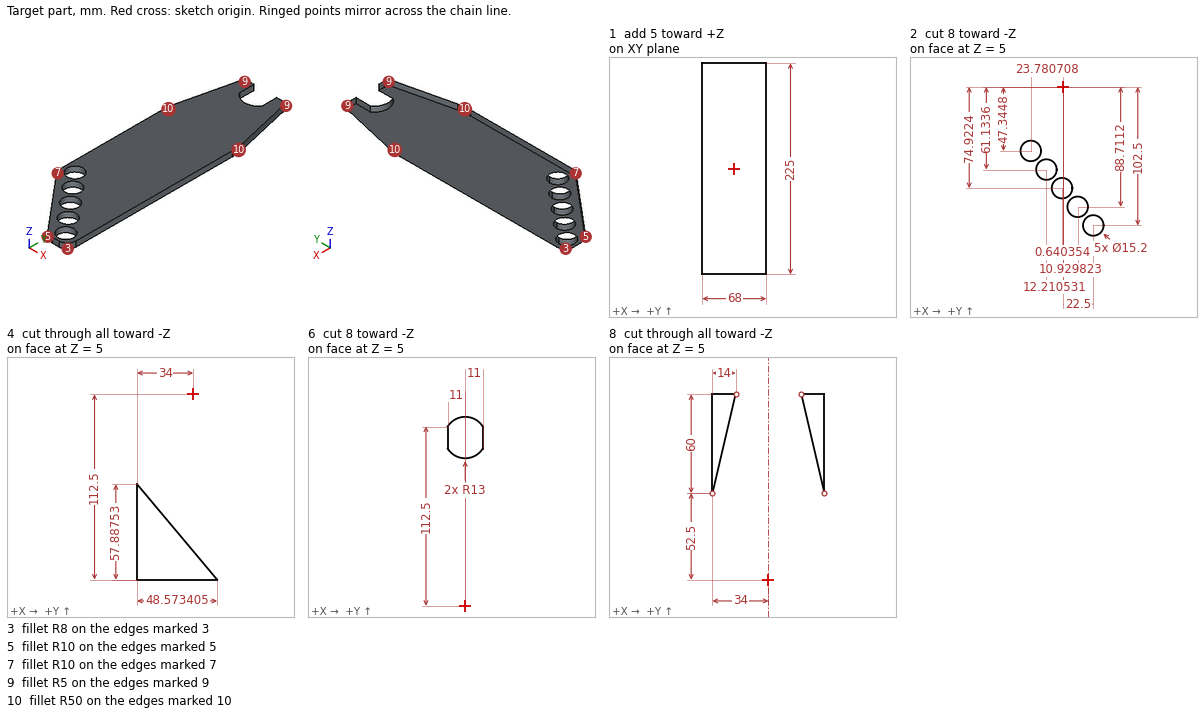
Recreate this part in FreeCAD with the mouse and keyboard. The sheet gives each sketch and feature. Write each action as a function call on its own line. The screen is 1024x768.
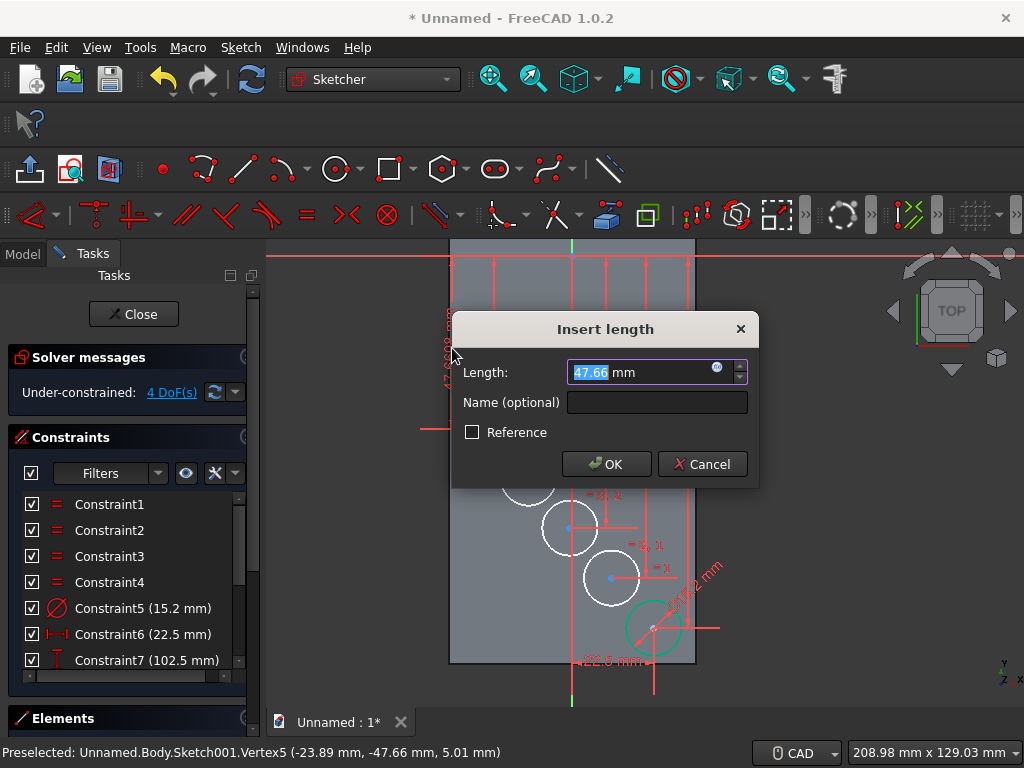
text(47.3448)
key(Return)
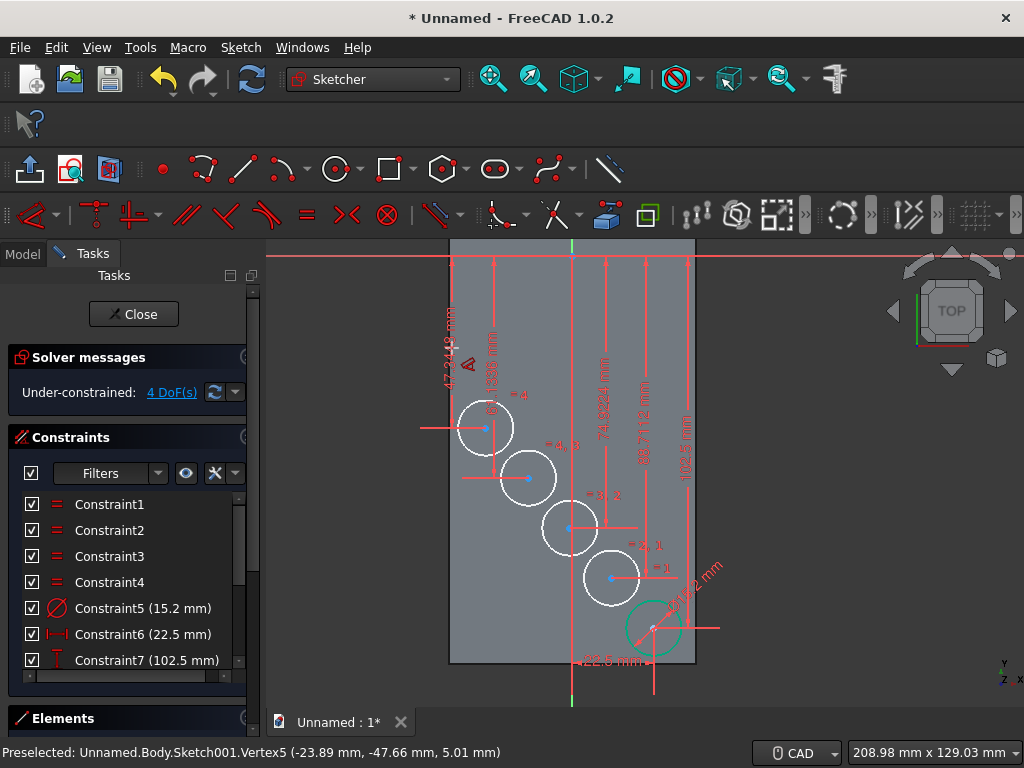
scroll(570, 528, up, 15)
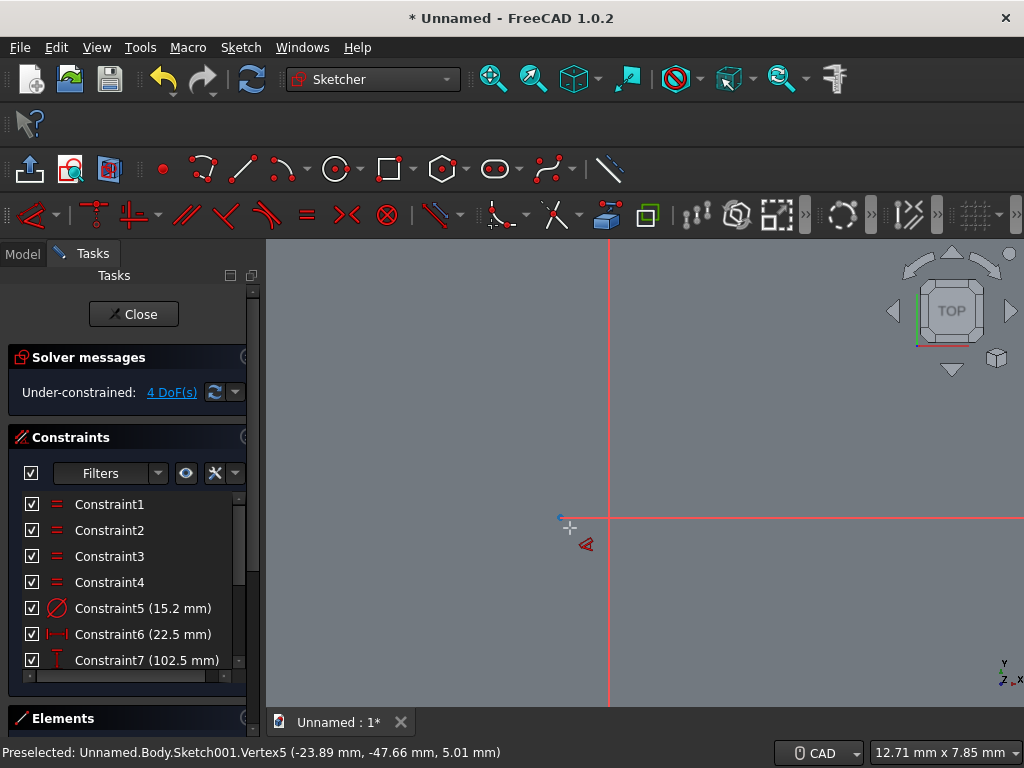
click(561, 518)
click(585, 552)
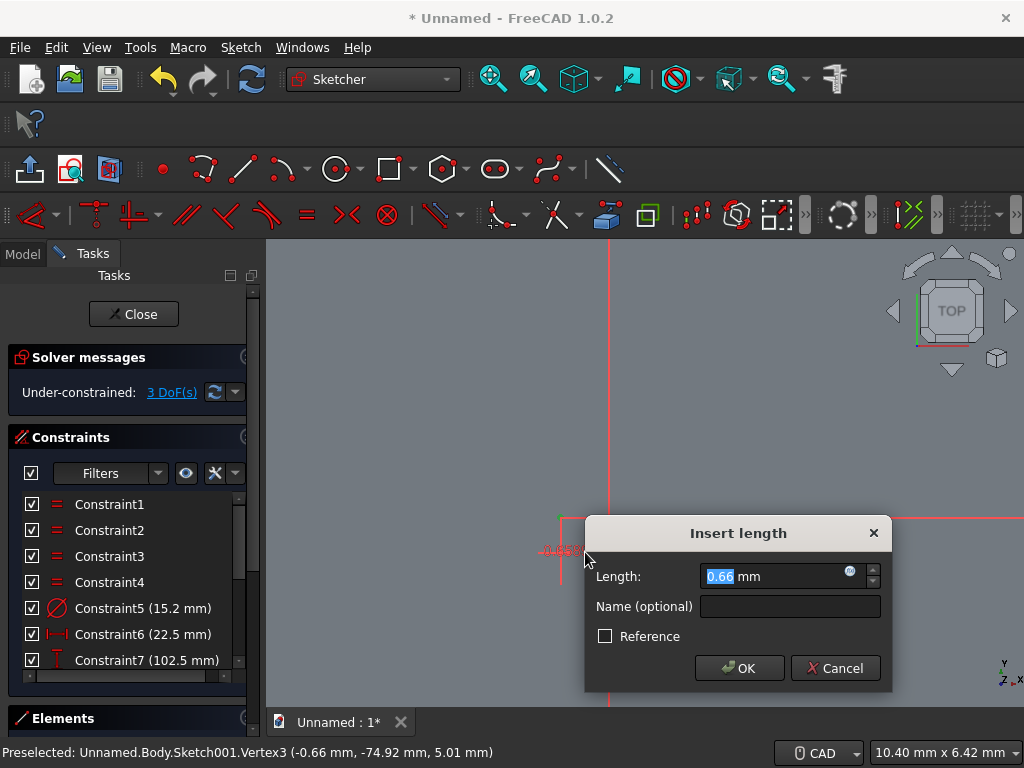
text(0.640354)
key(Return)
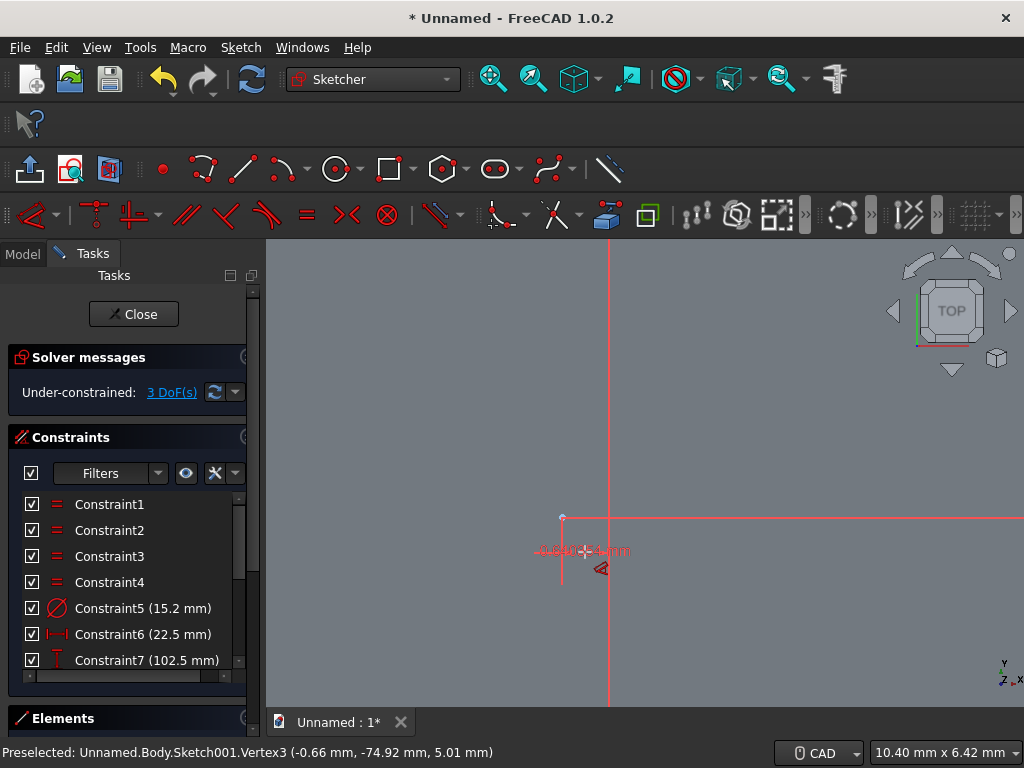
scroll(577, 533, down, 16)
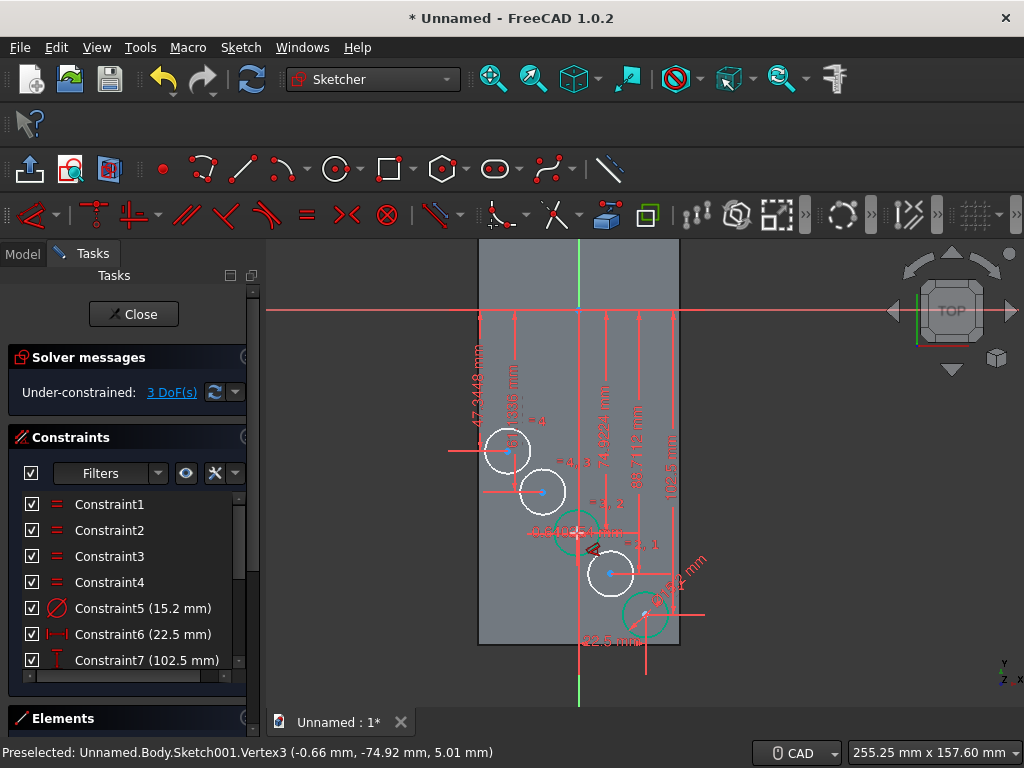
scroll(611, 574, up, 2)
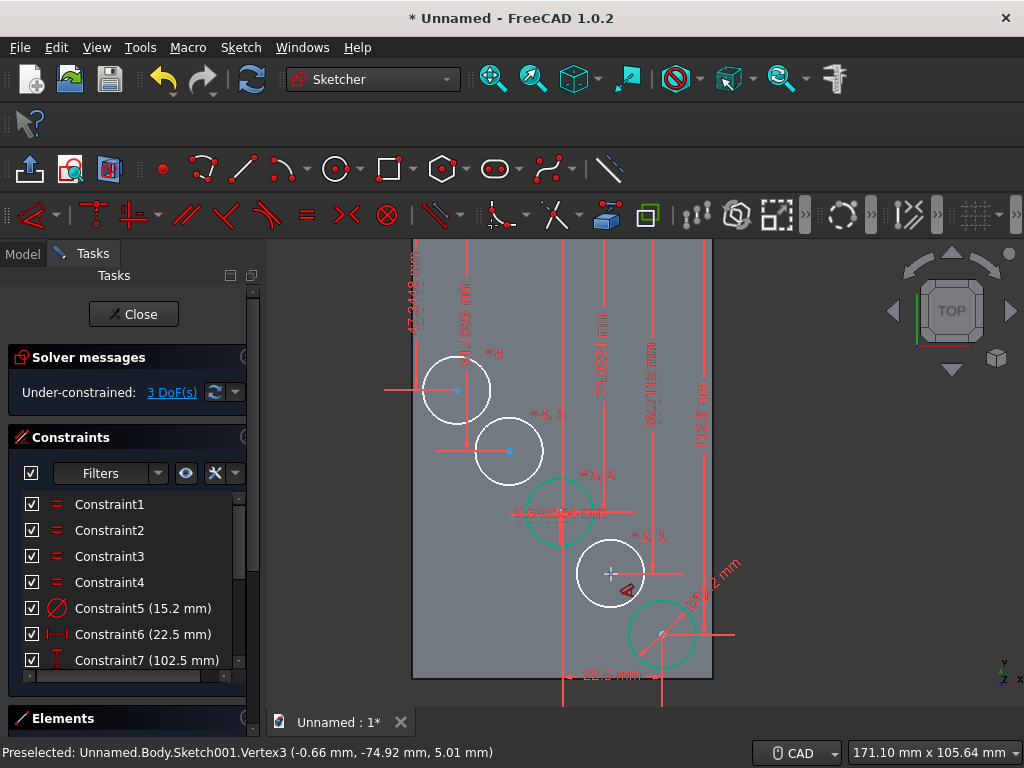
click(611, 574)
click(587, 632)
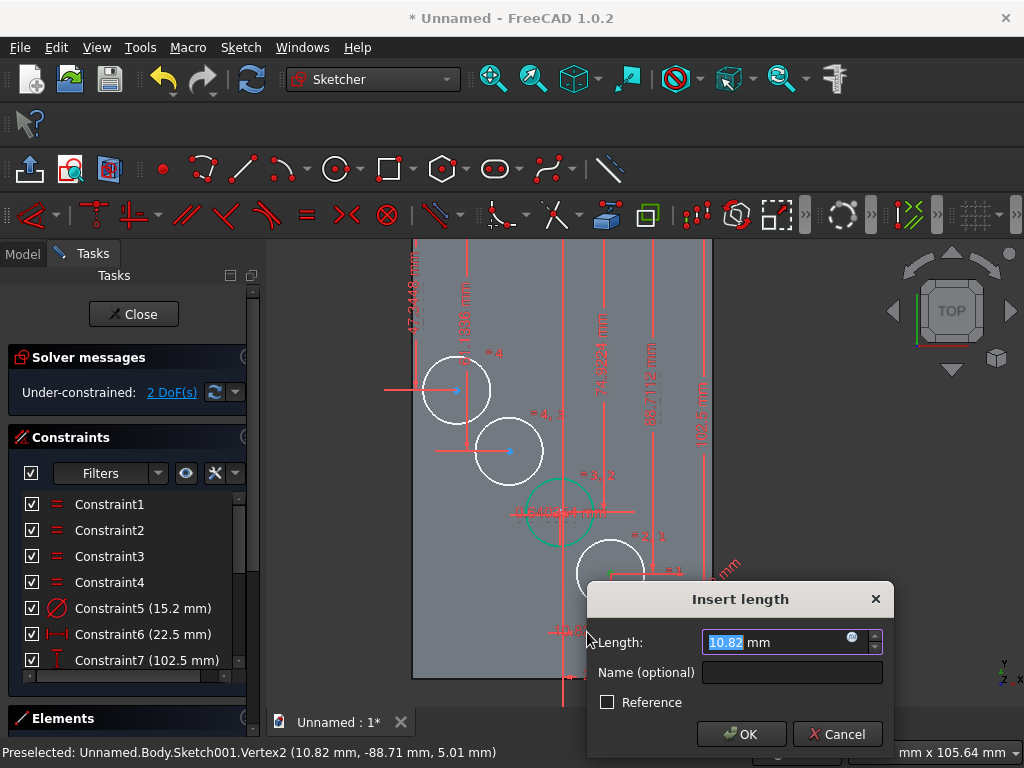
text(10.929823)
key(Return)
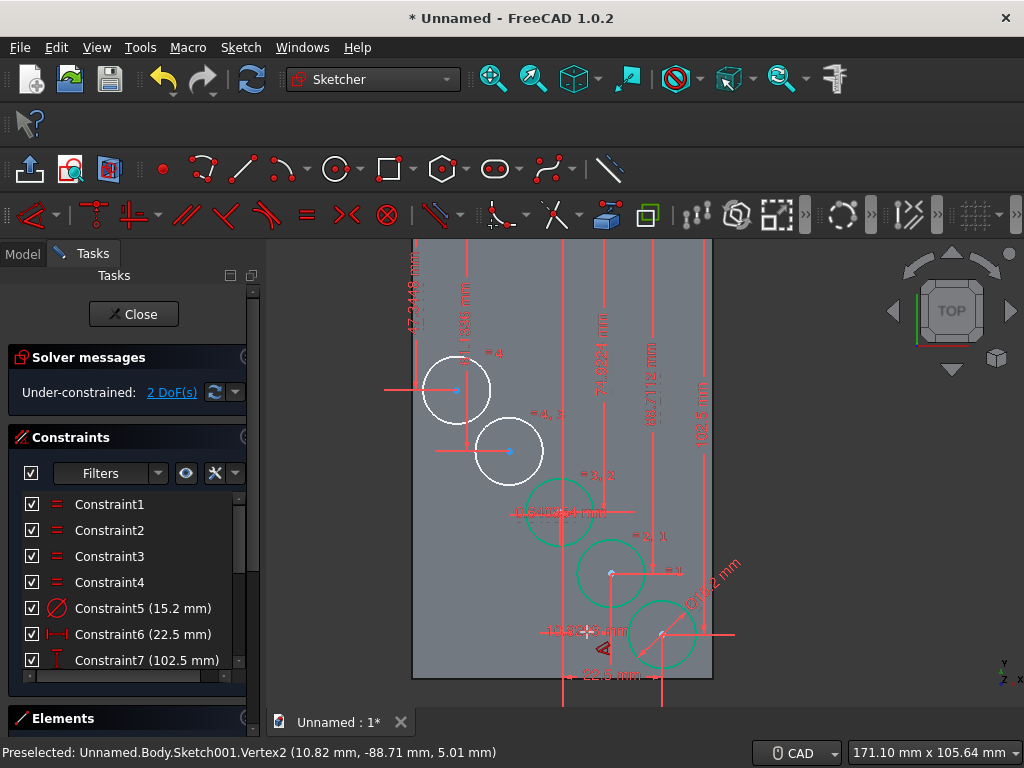
click(509, 451)
click(536, 557)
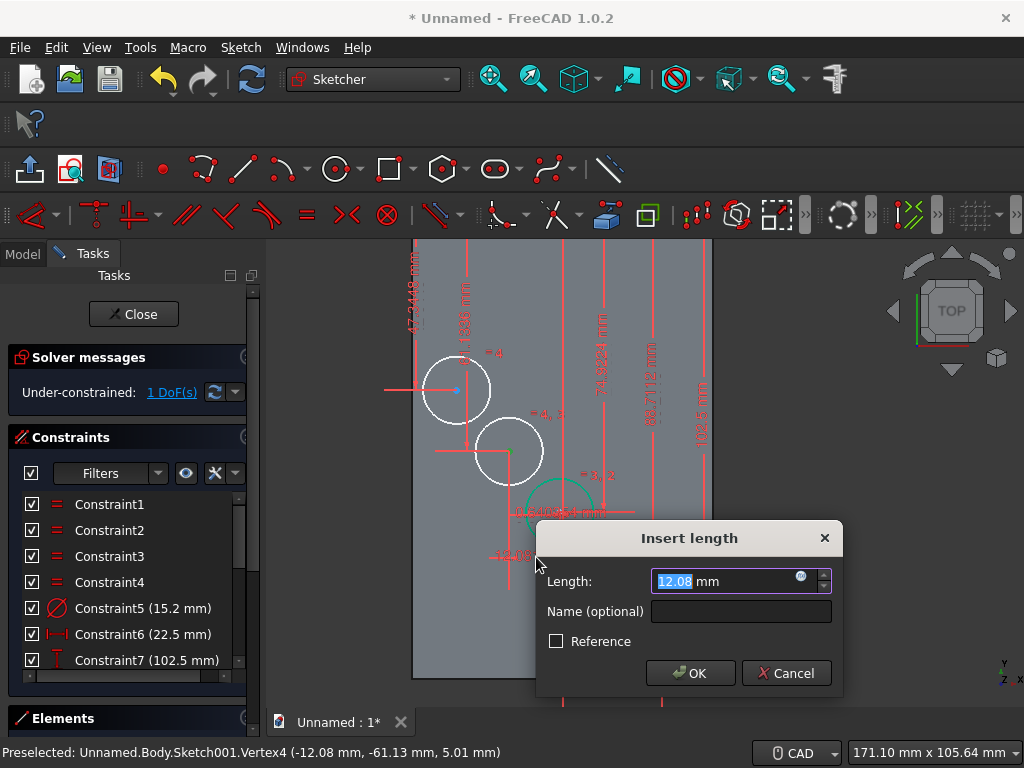
text(12.210531)
key(Return)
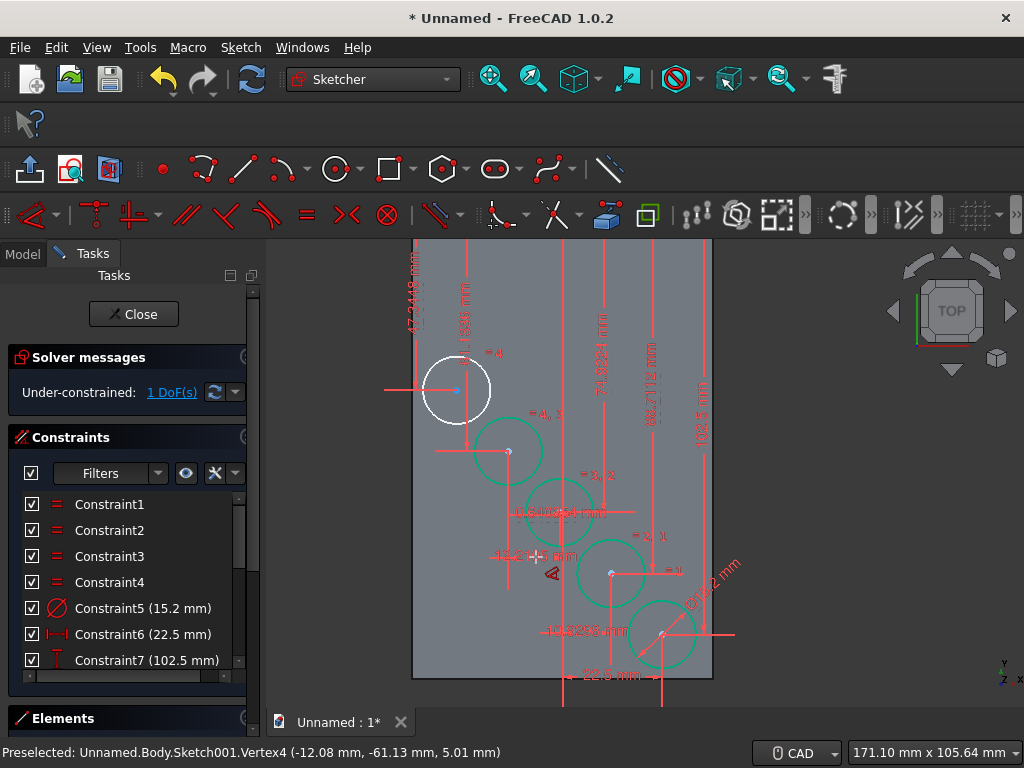
click(457, 390)
click(547, 424)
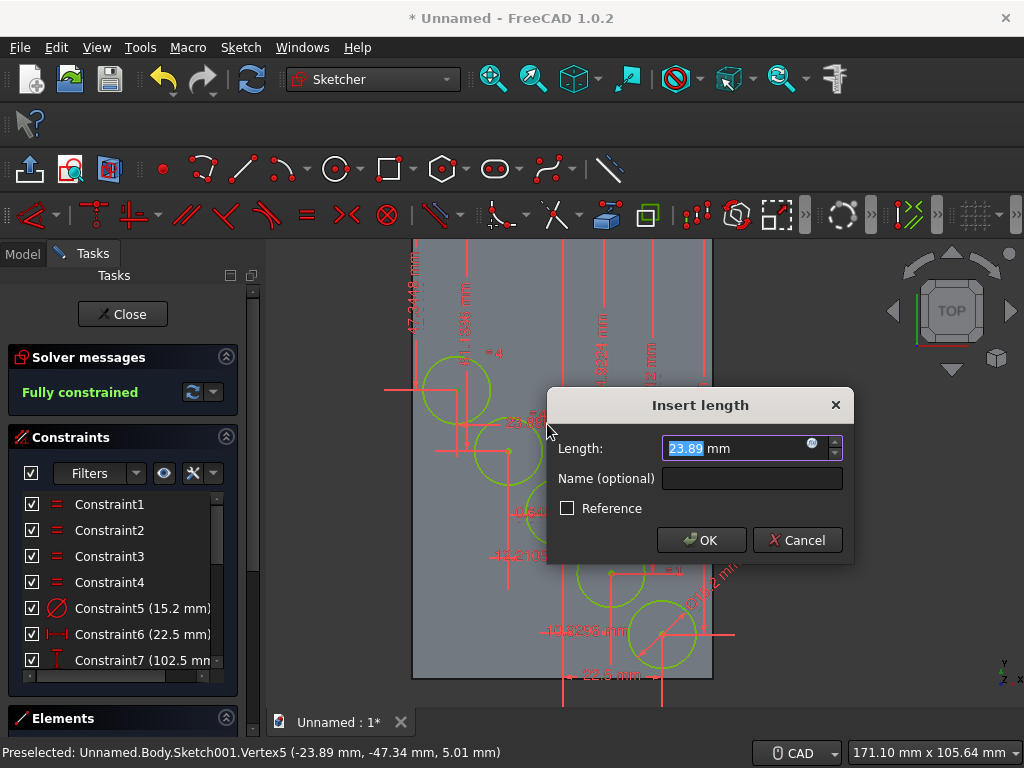
text(23.780708)
key(Return)
key(Escape)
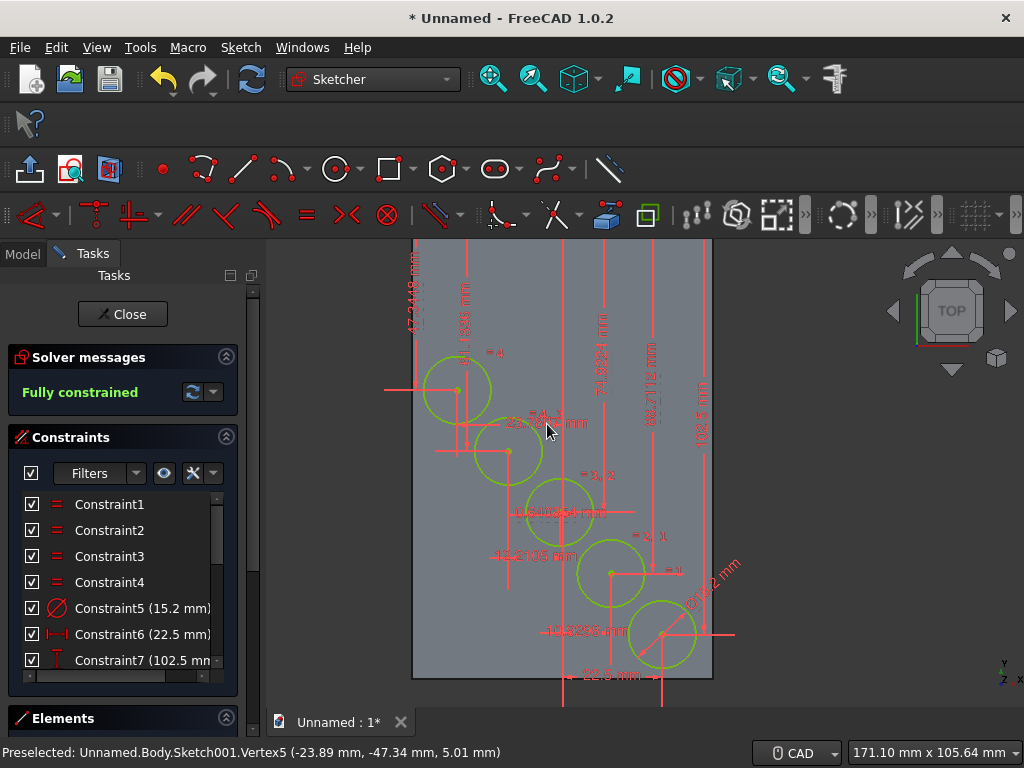
click(123, 314)